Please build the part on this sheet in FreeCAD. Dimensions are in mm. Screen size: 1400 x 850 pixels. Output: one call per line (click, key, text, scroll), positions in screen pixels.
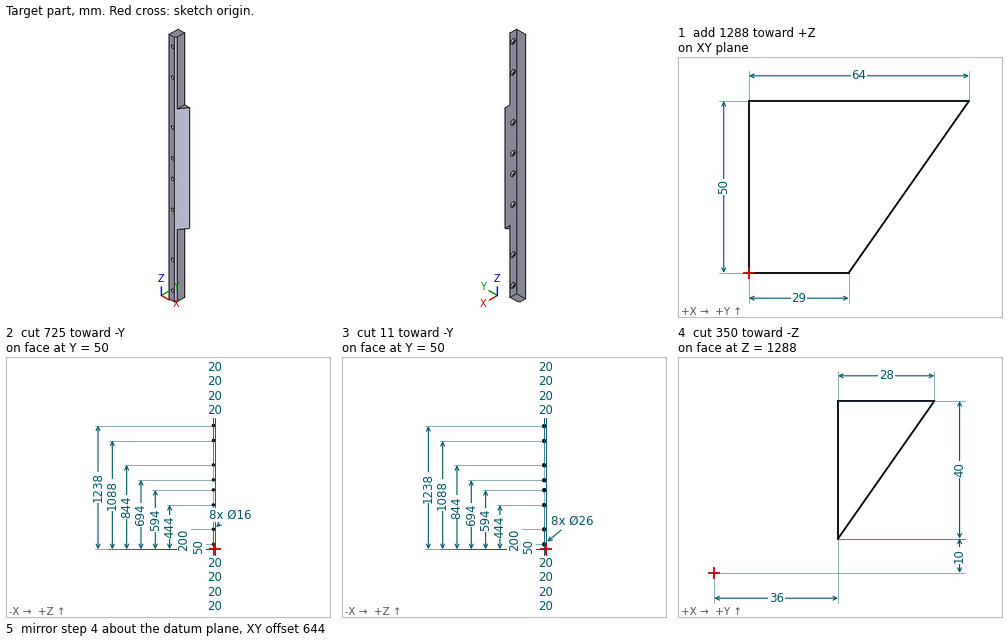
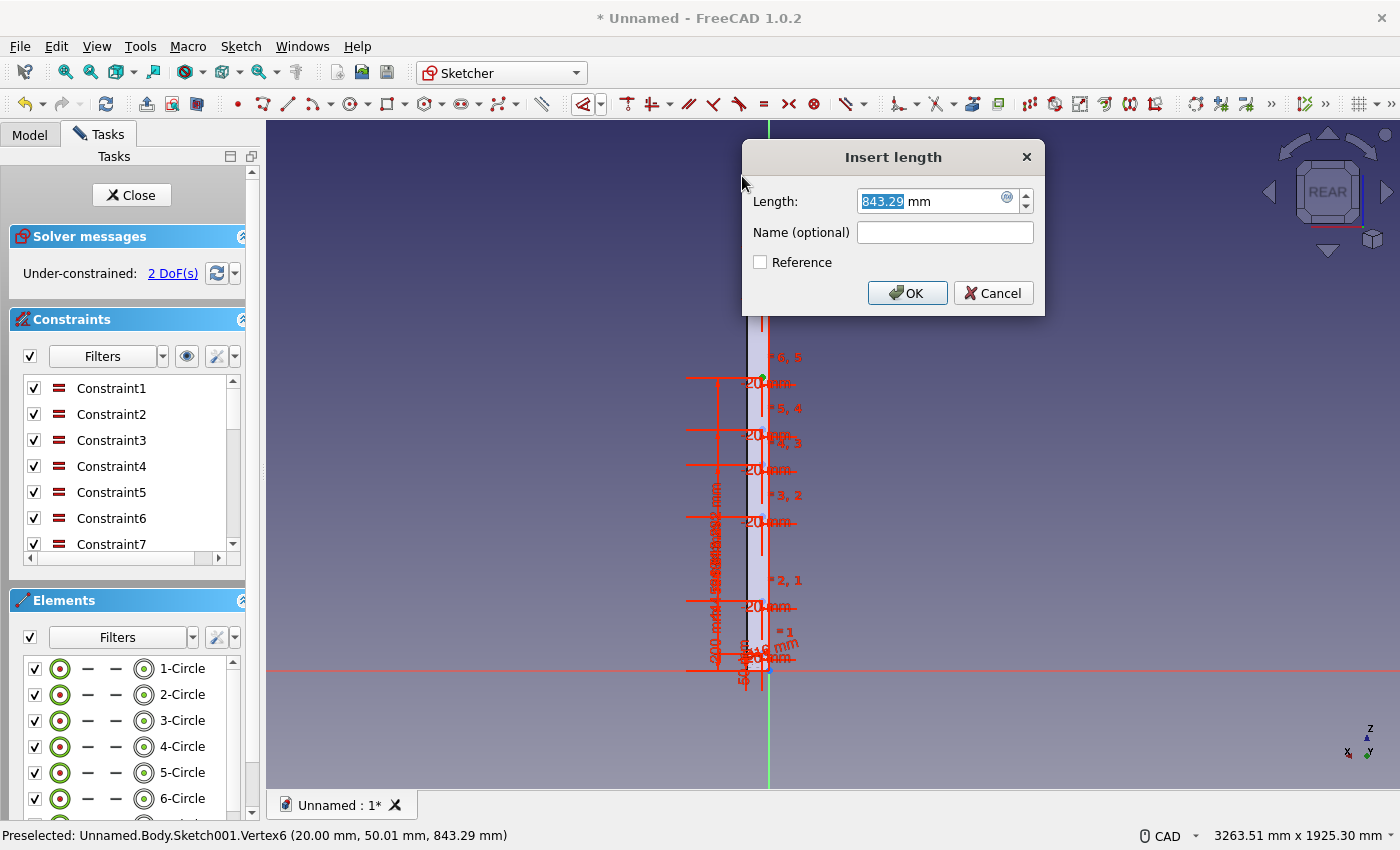
text(844)
key(Return)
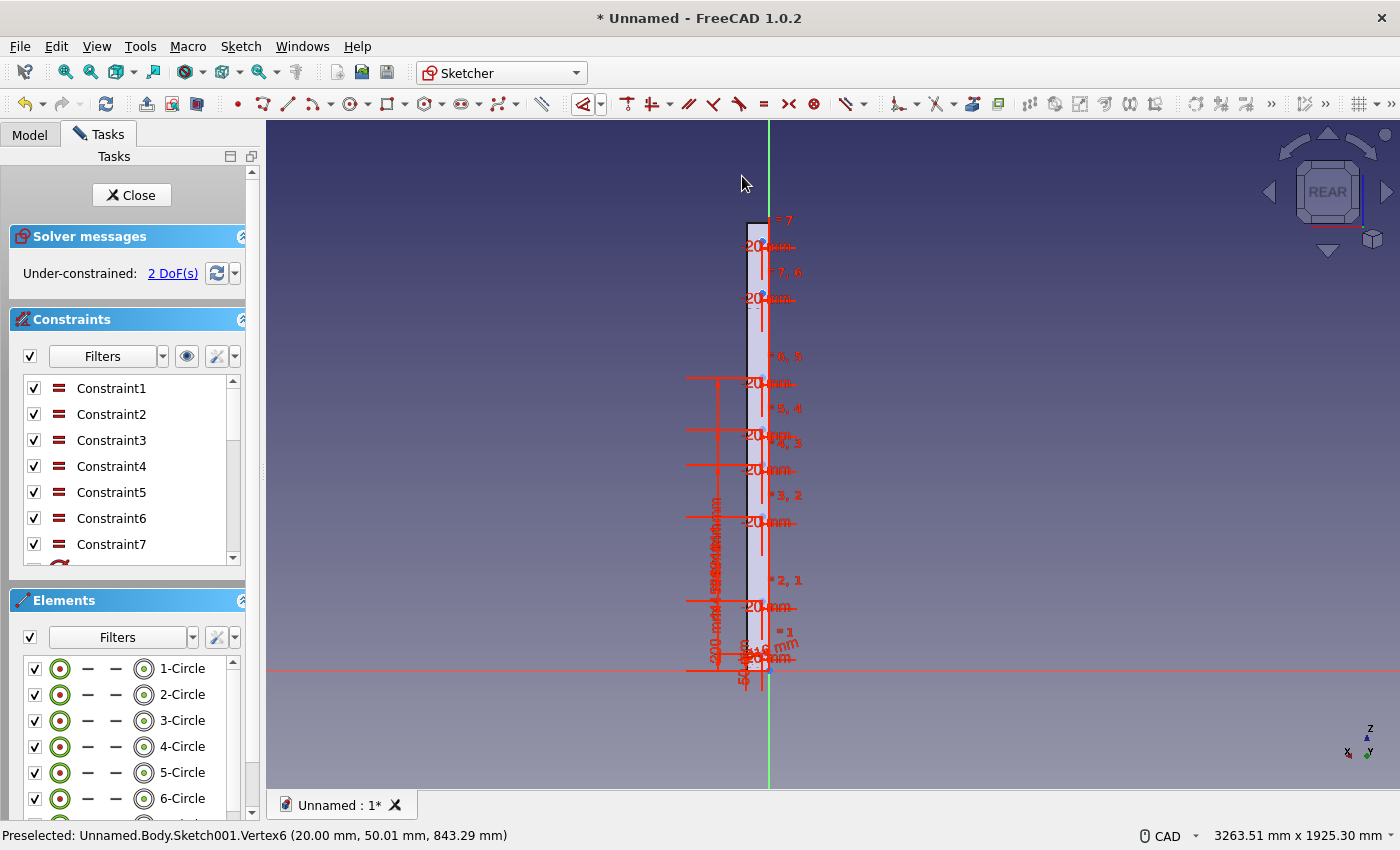
click(762, 293)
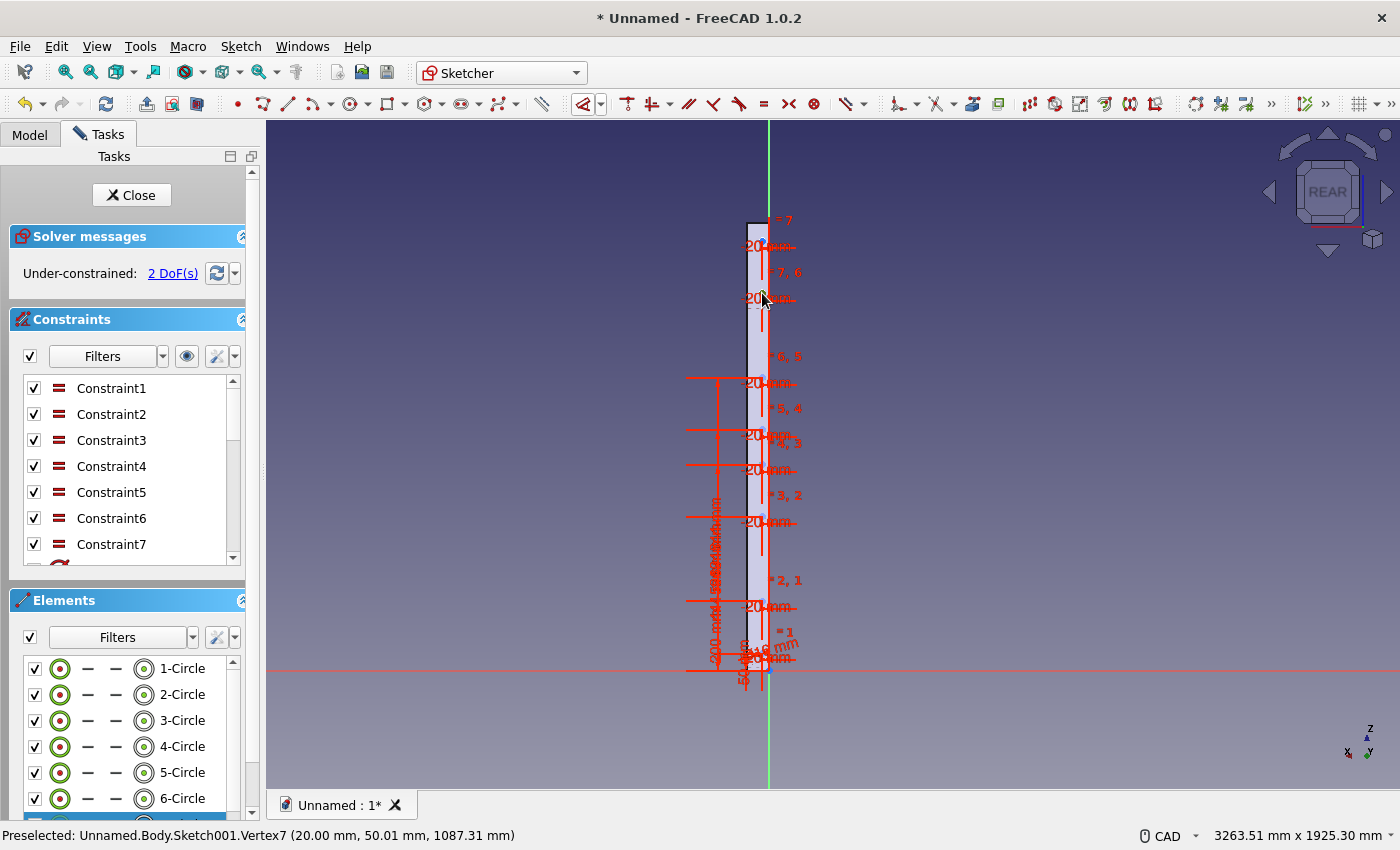
key(i)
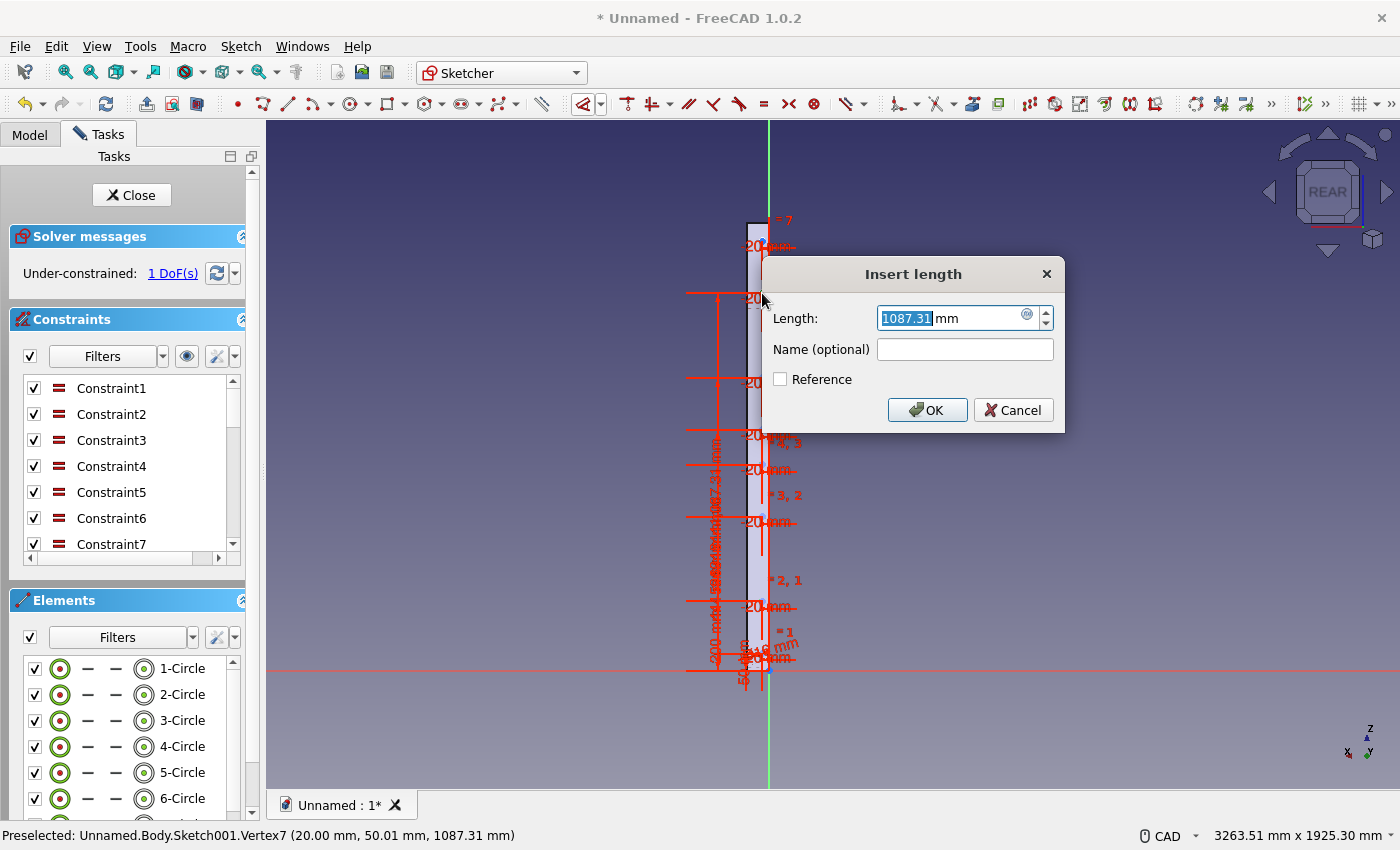
text(1088)
key(Return)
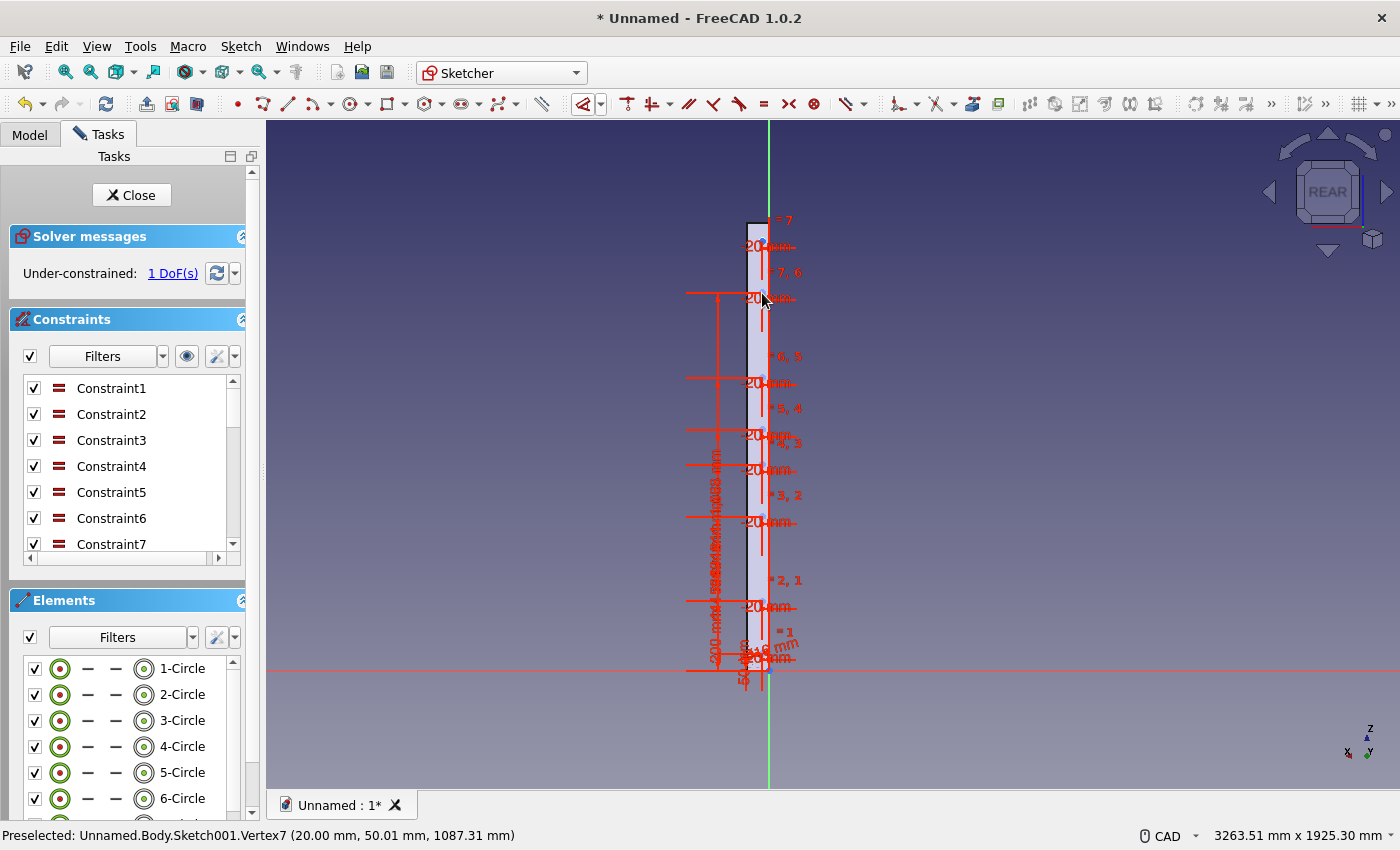
click(762, 241)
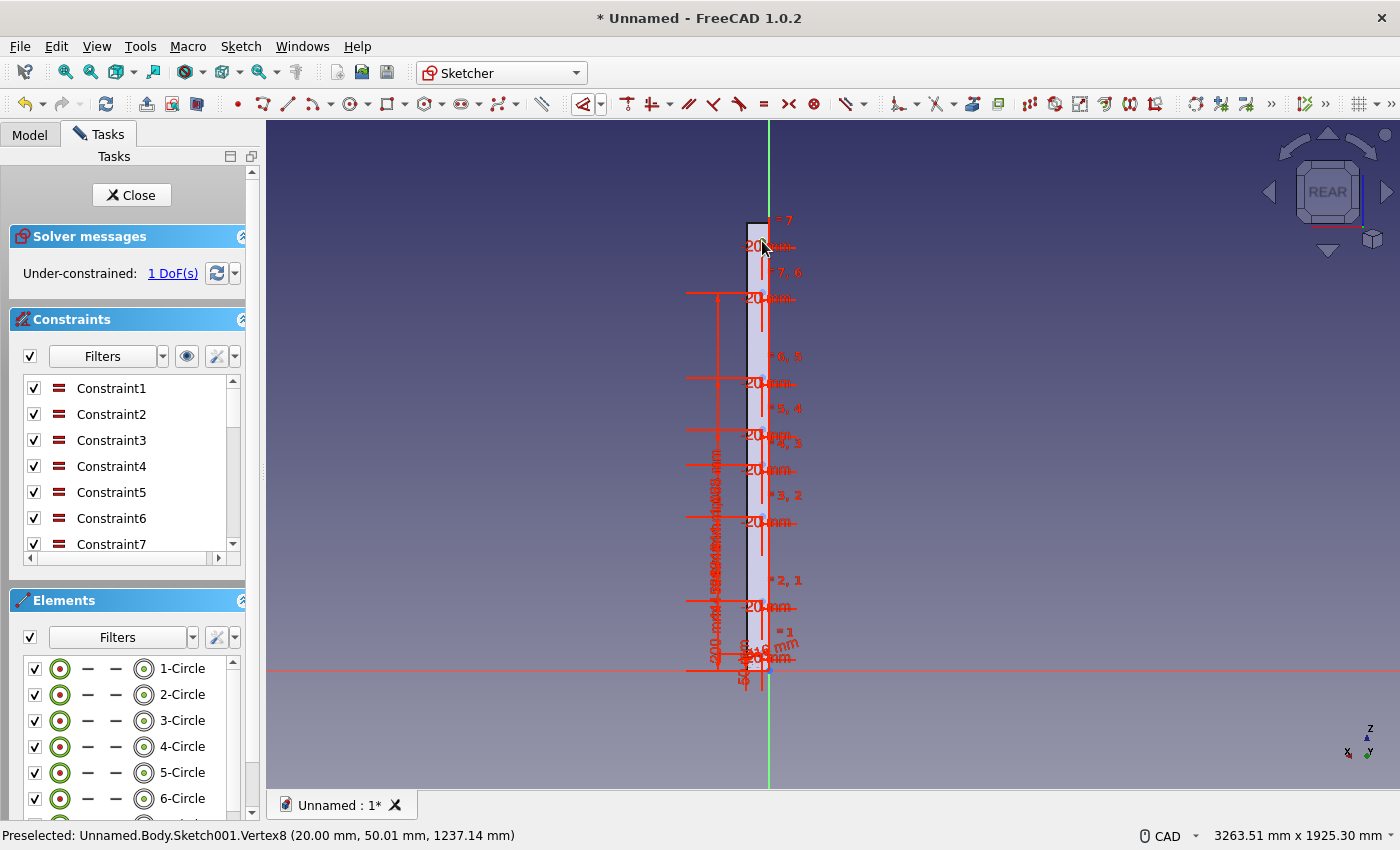
key(i)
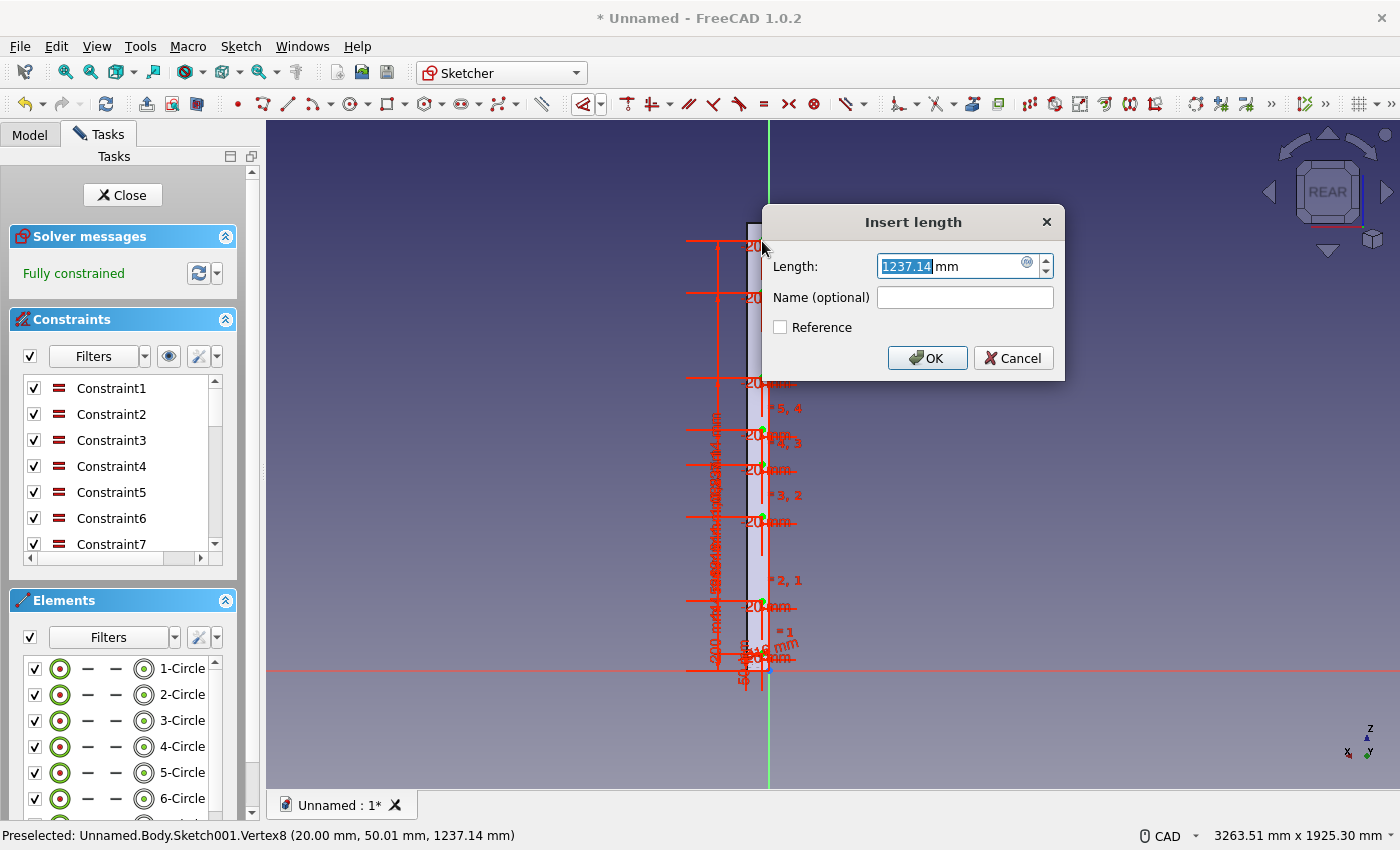
text(1238)
key(Return)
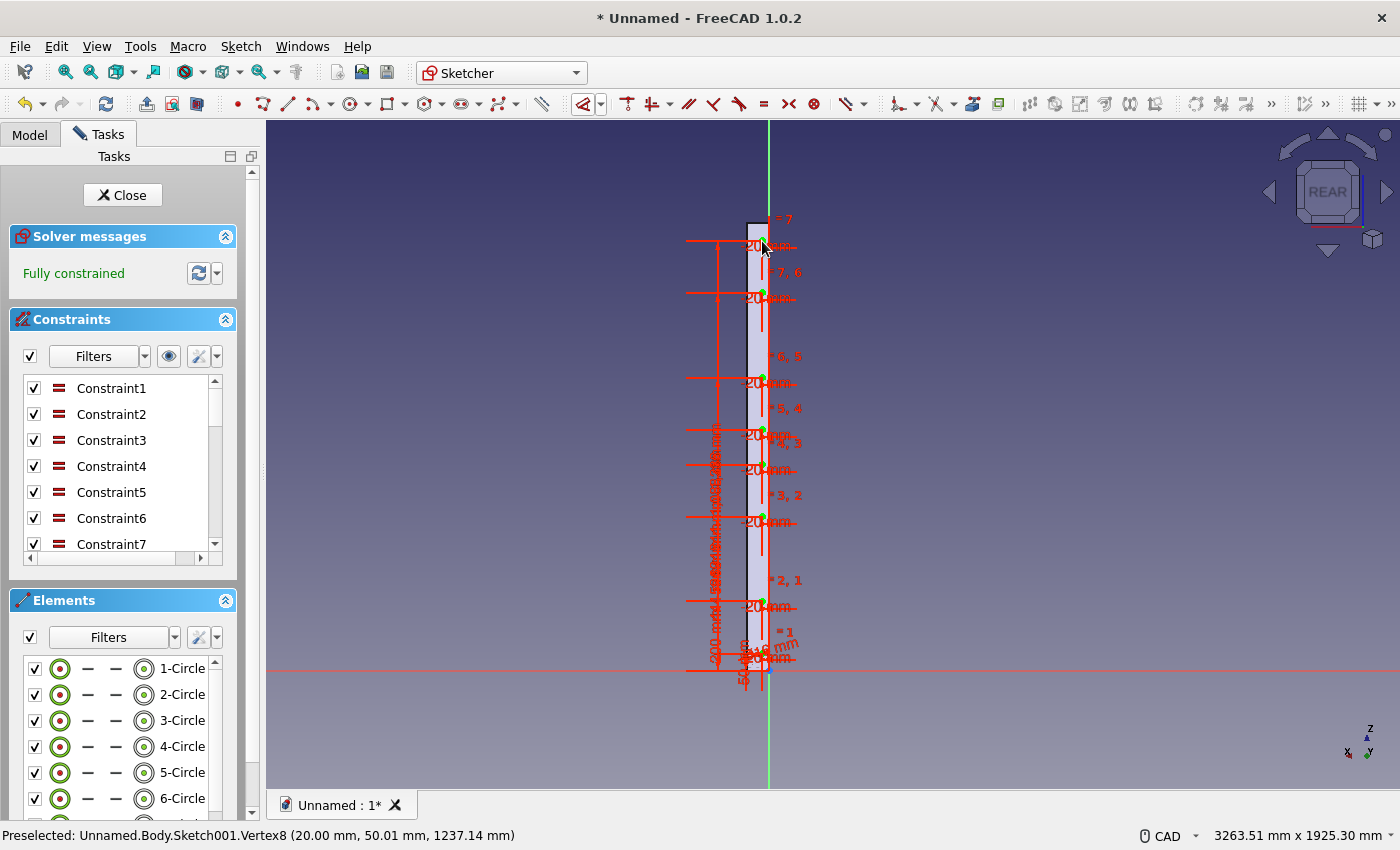
click(123, 195)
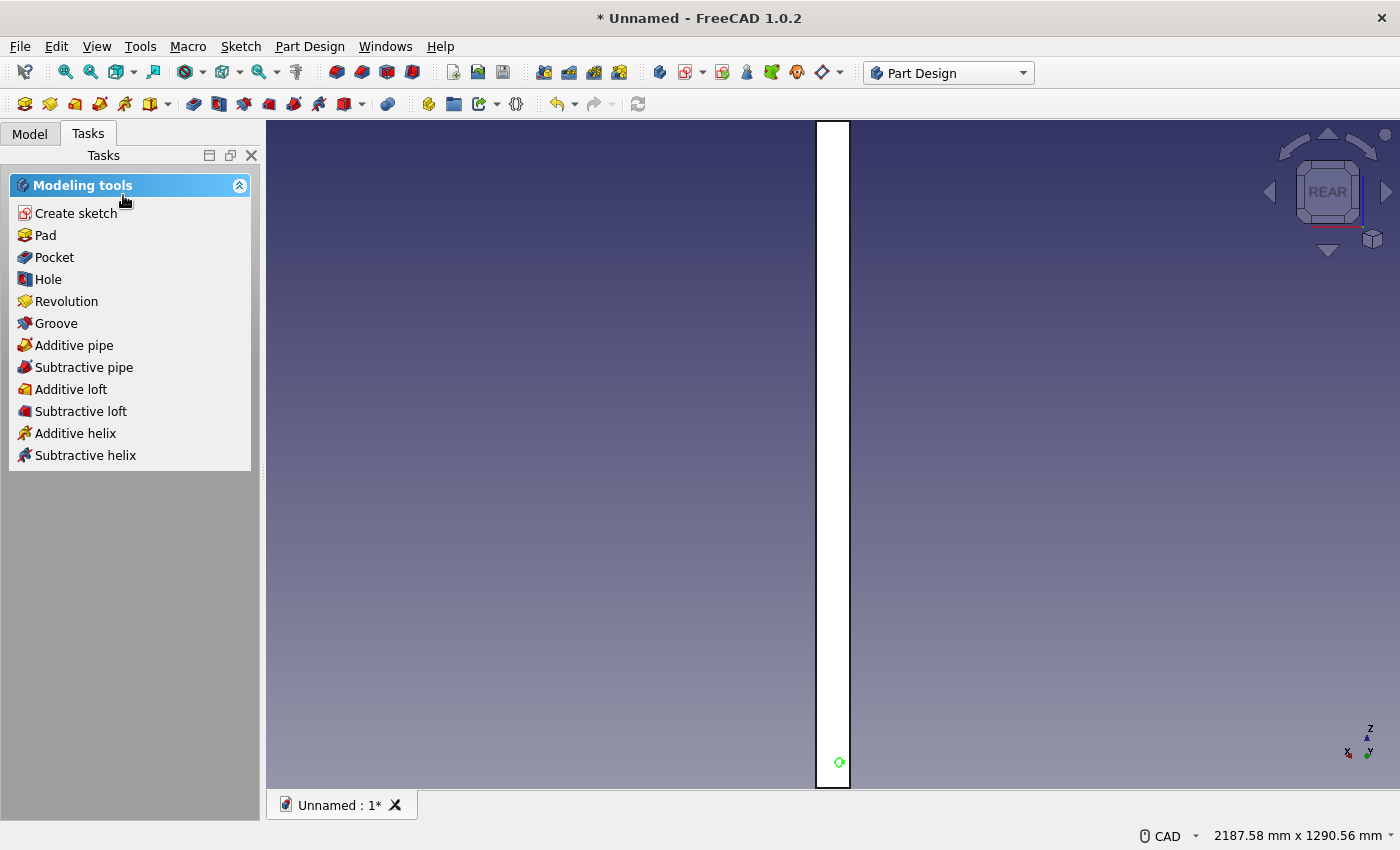
click(194, 104)